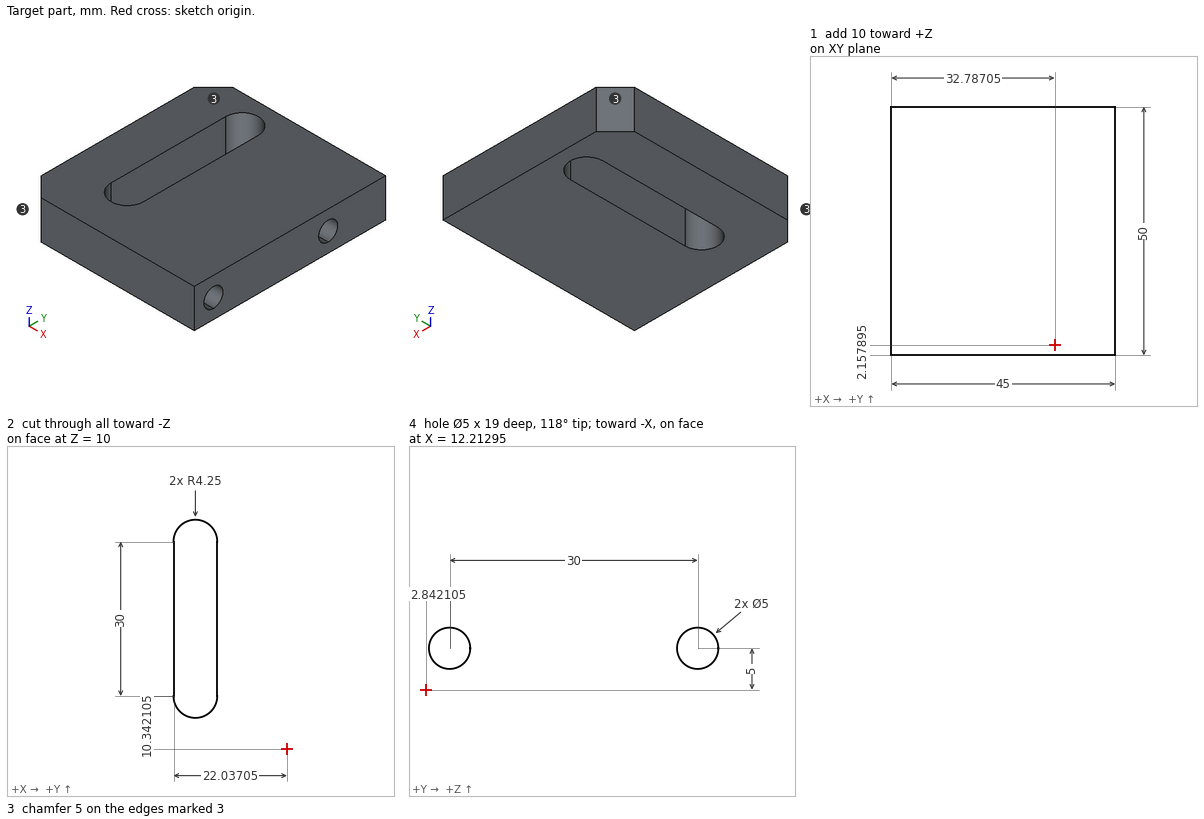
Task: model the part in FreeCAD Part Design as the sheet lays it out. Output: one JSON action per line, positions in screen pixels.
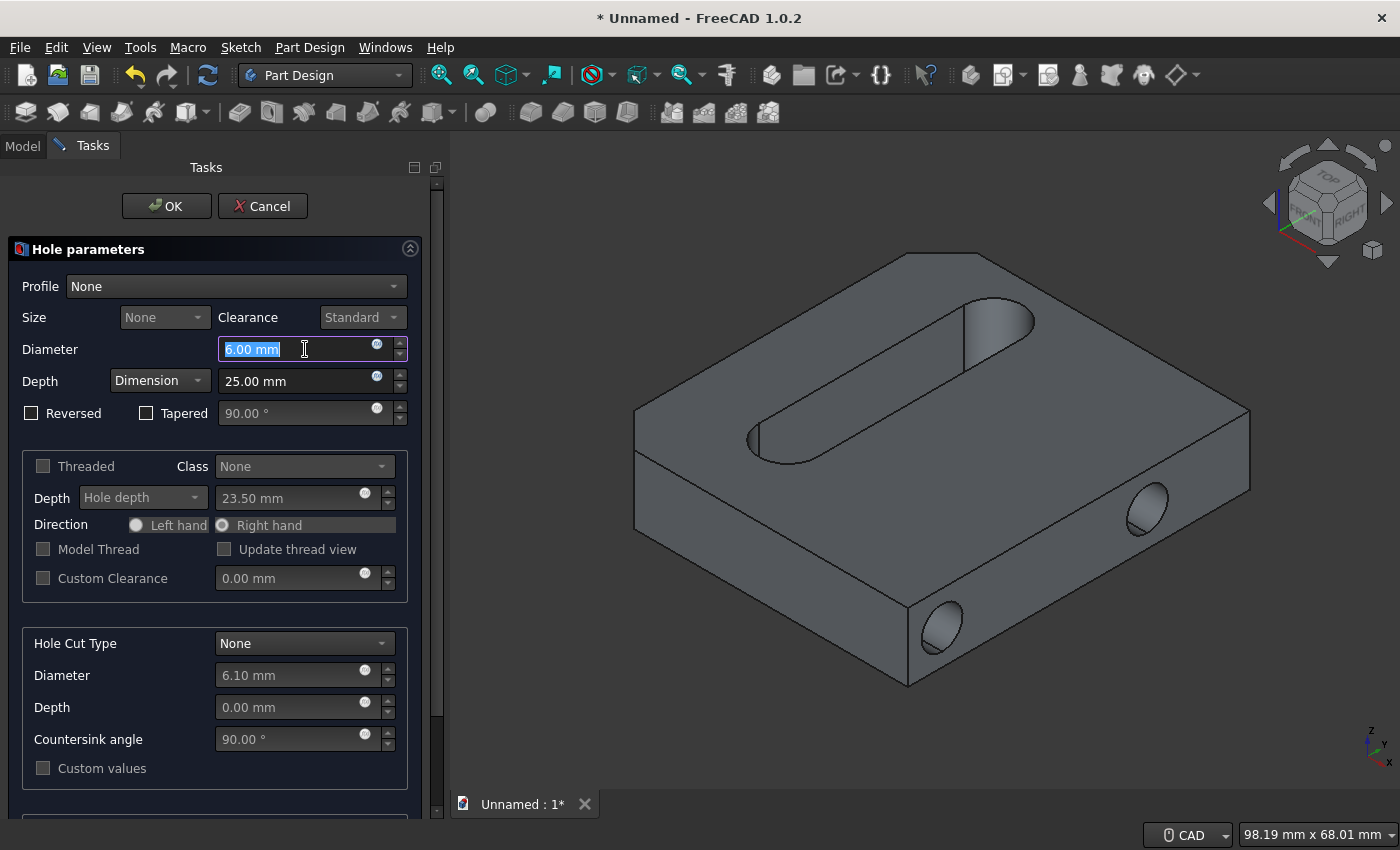
{"action": "type", "text": "5"}
{"action": "key", "text": "Tab"}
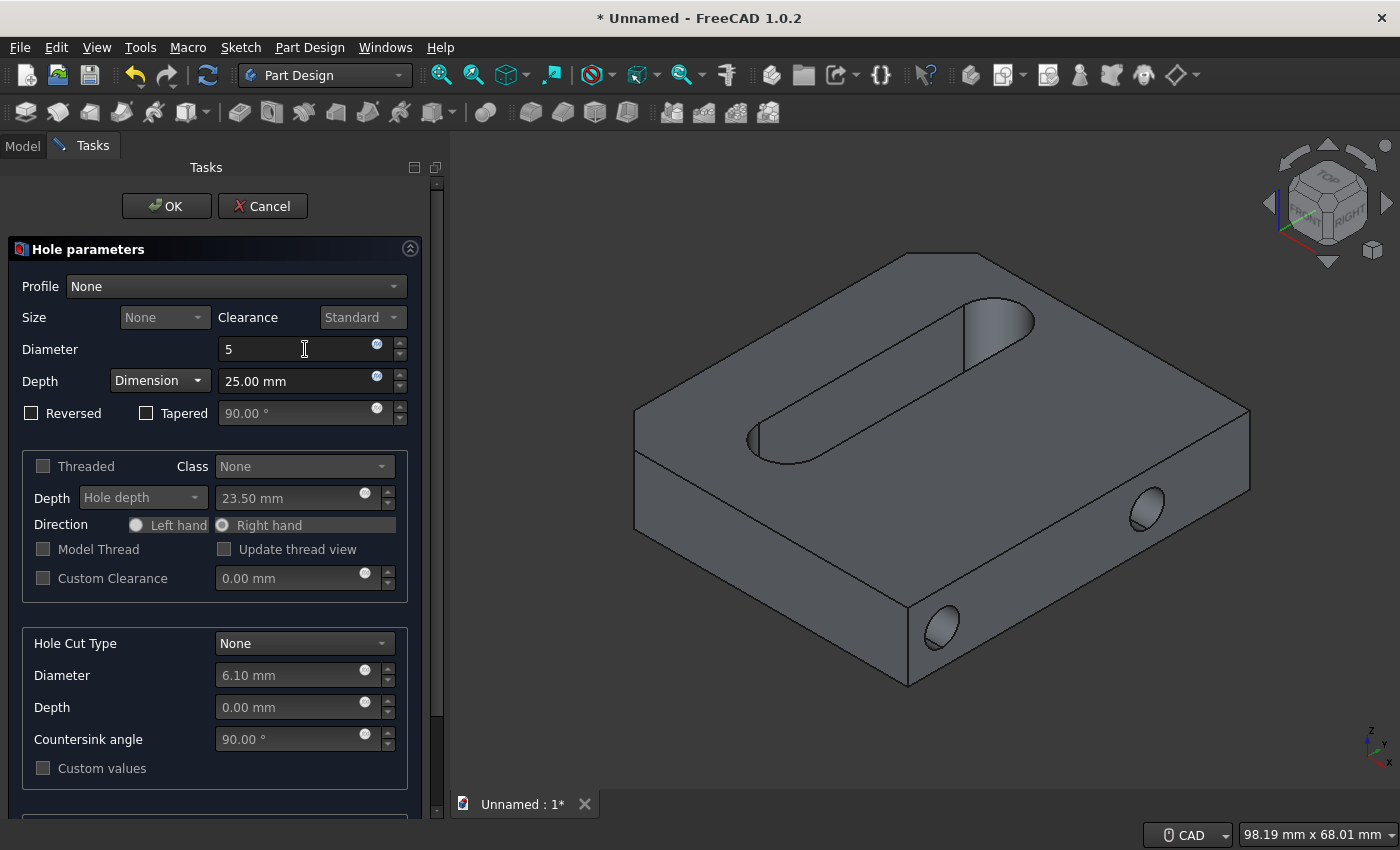
{"action": "triple_click", "coordinate": [305, 381]}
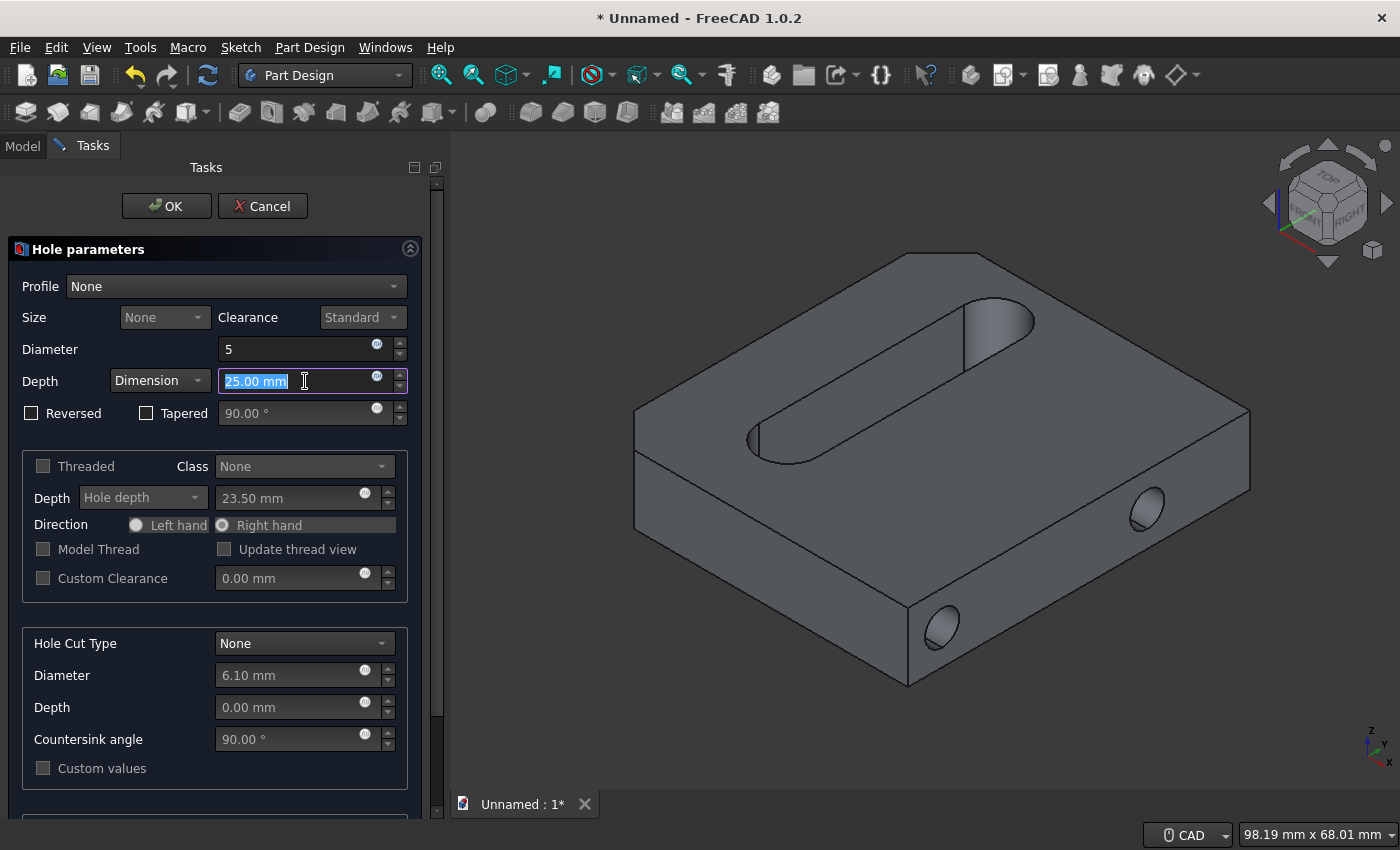
{"action": "type", "text": "19"}
{"action": "key", "text": "Tab"}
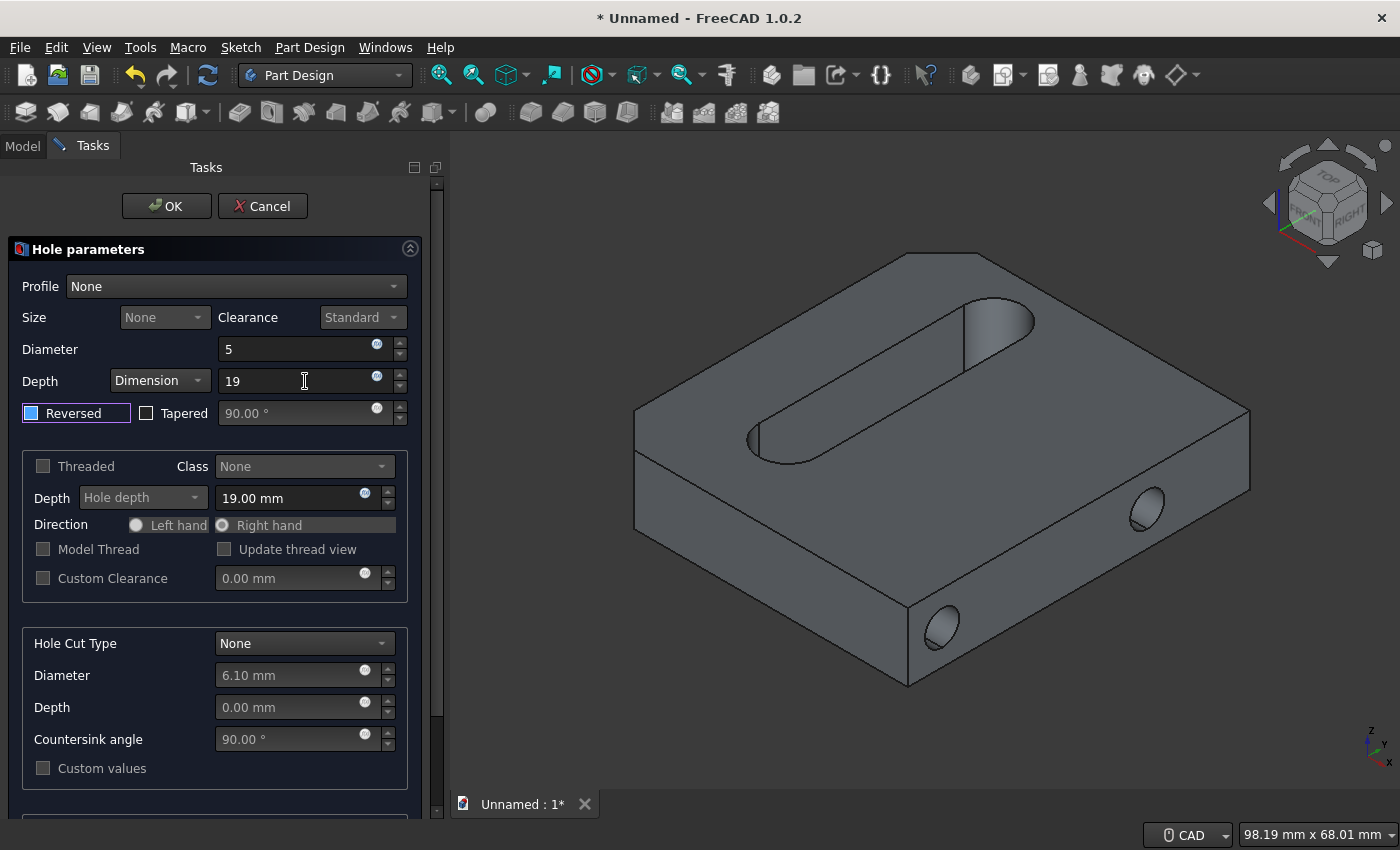
{"action": "left_click", "coordinate": [167, 206]}